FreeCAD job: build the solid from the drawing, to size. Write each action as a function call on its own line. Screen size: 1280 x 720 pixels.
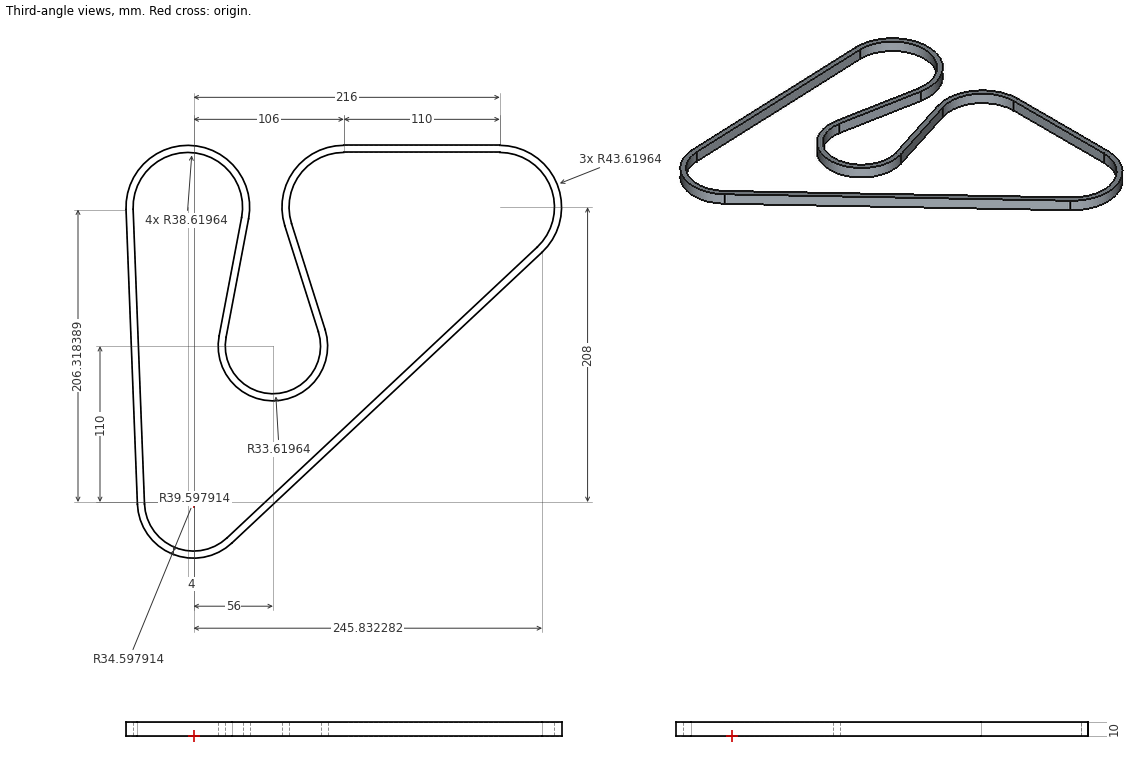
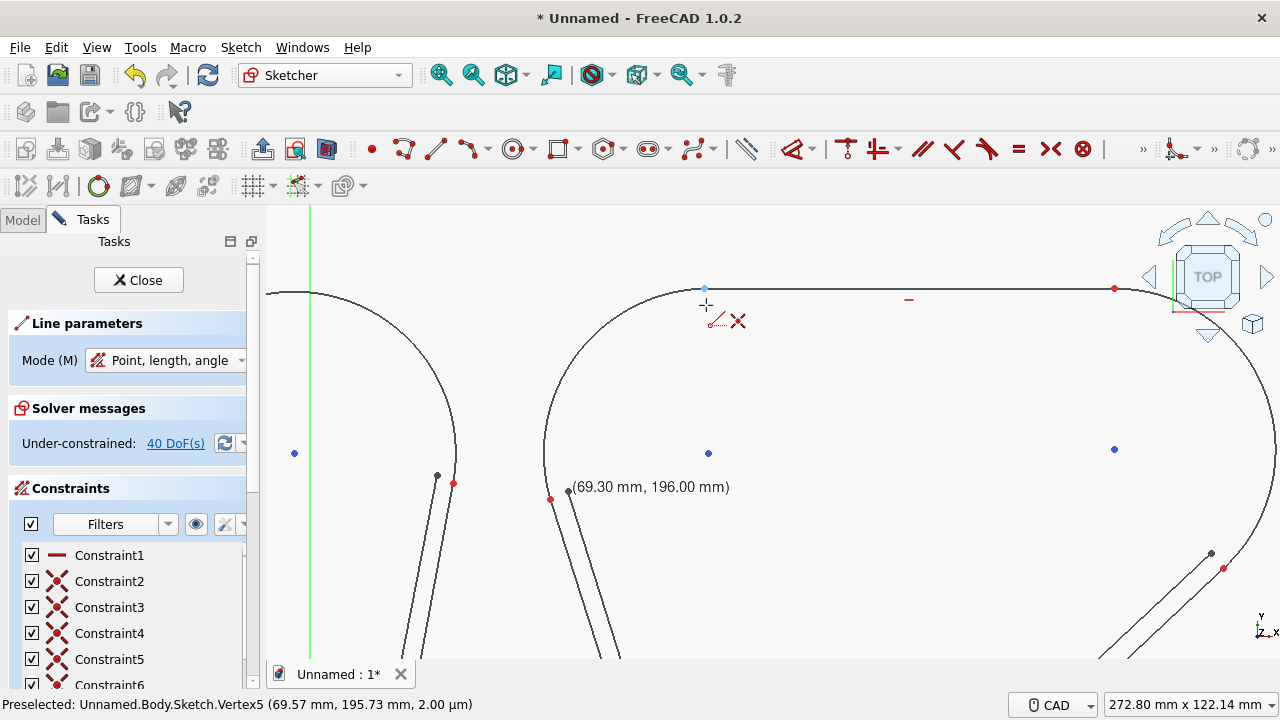
click(704, 304)
click(1113, 304)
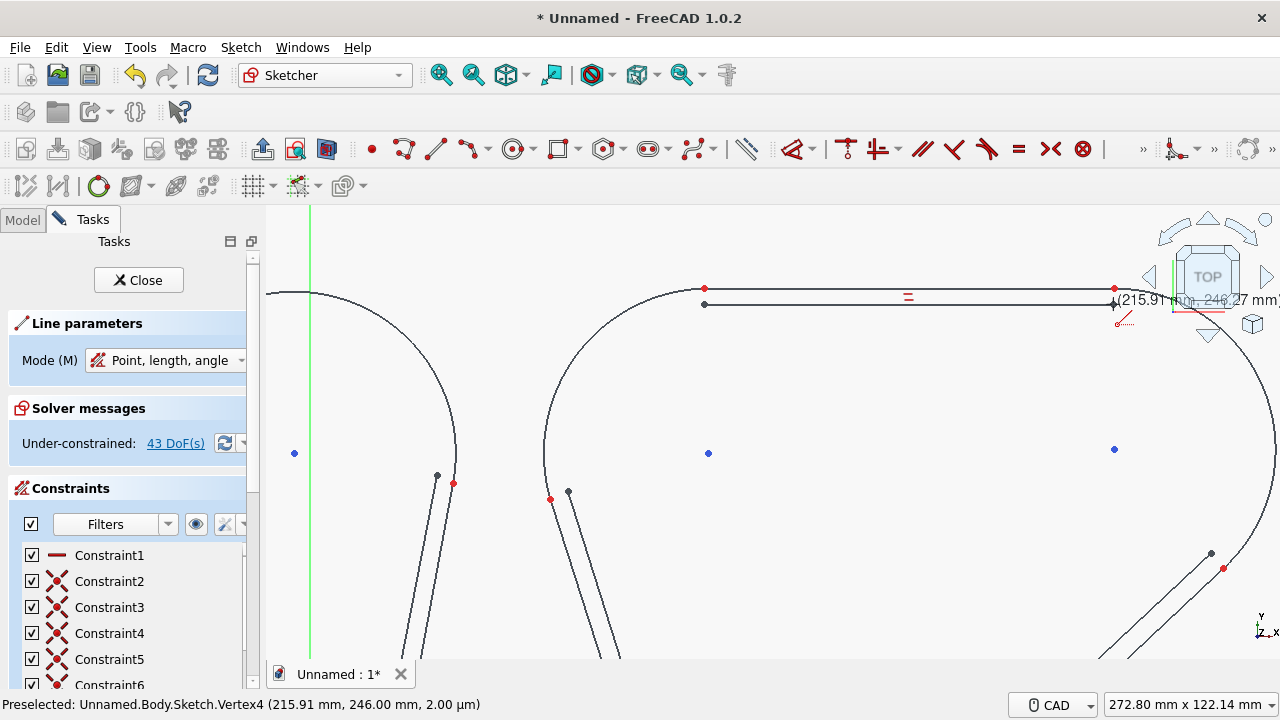
key(g)
key(3)
key(a)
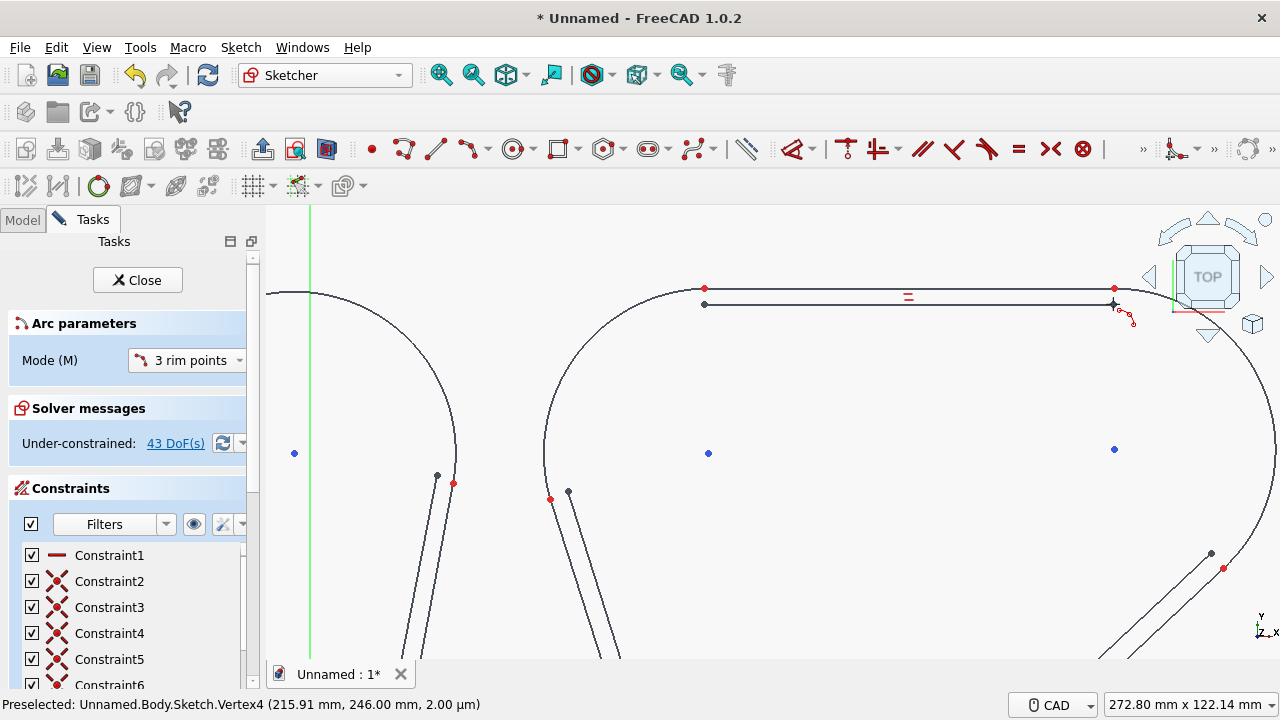
scroll(706, 305, down, 7)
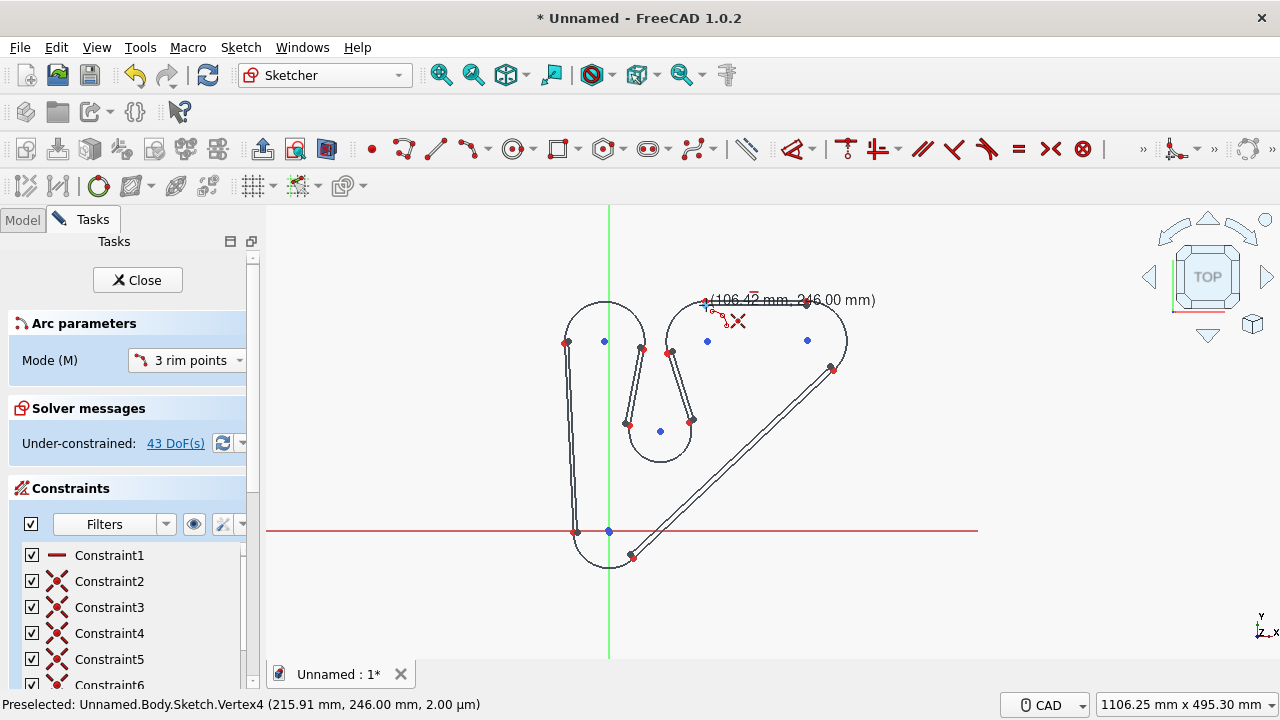
scroll(630, 554, up, 7)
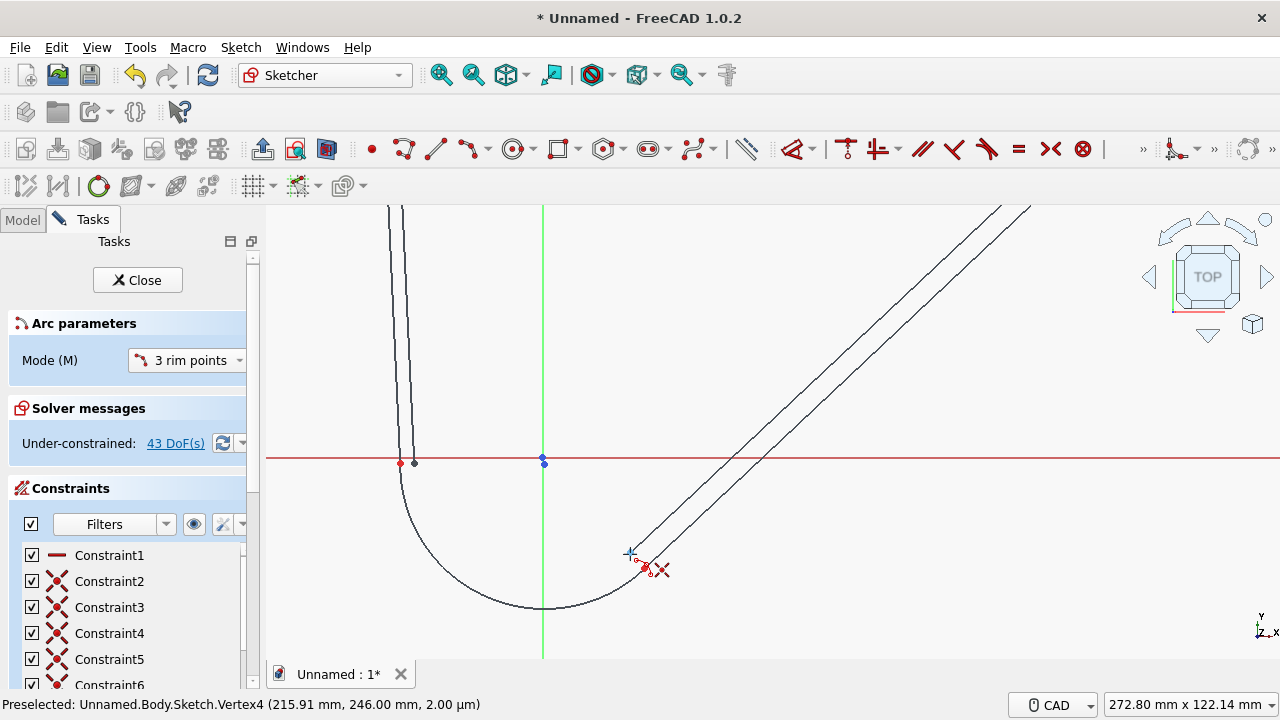
click(631, 552)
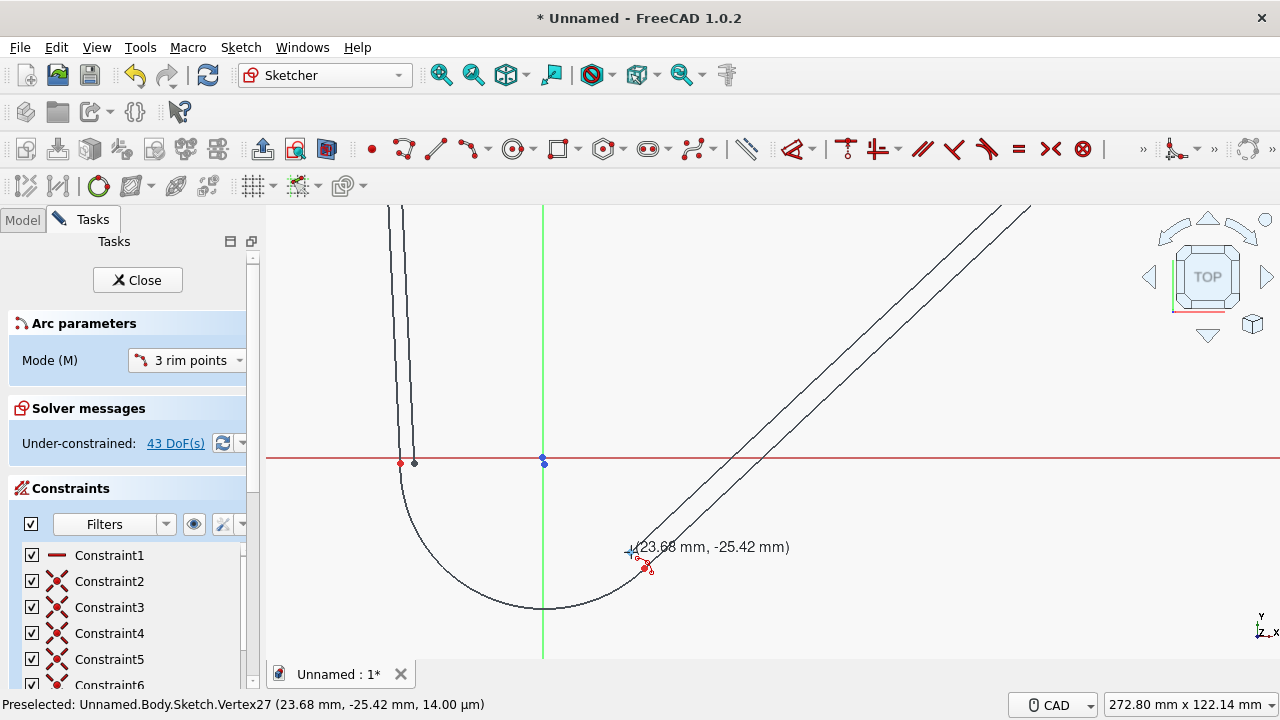
scroll(414, 463, up, 6)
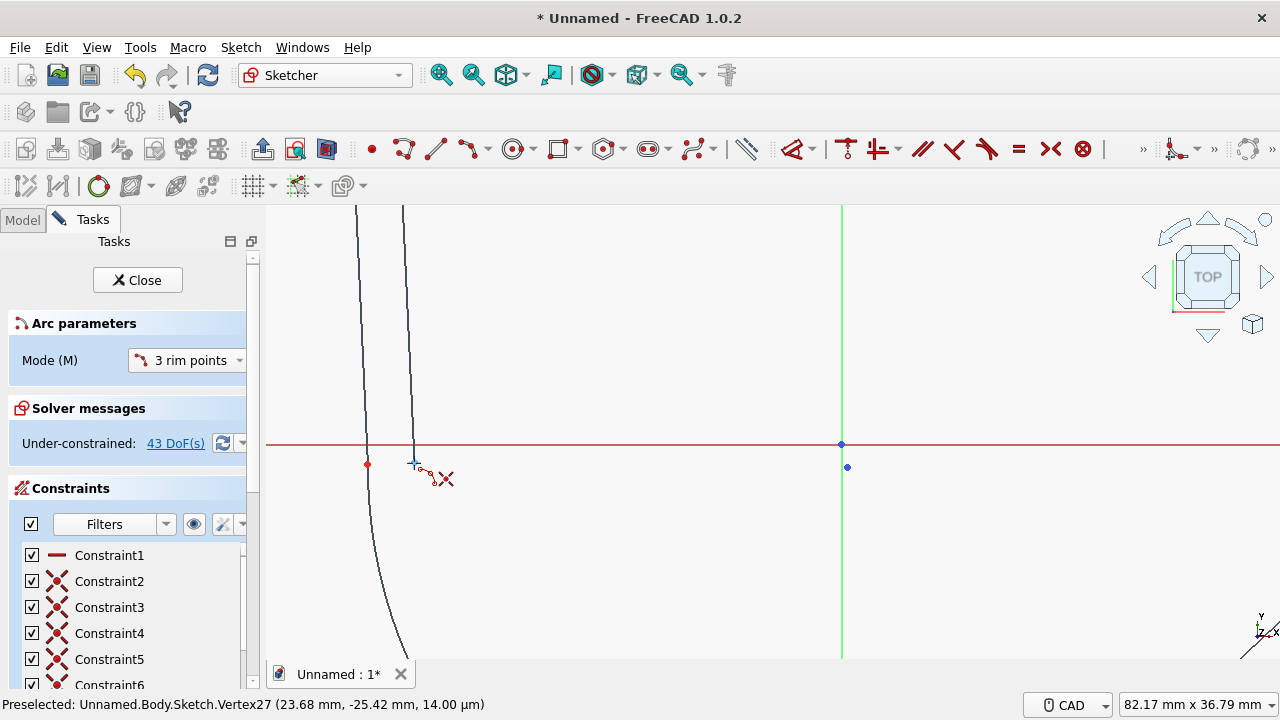
click(415, 462)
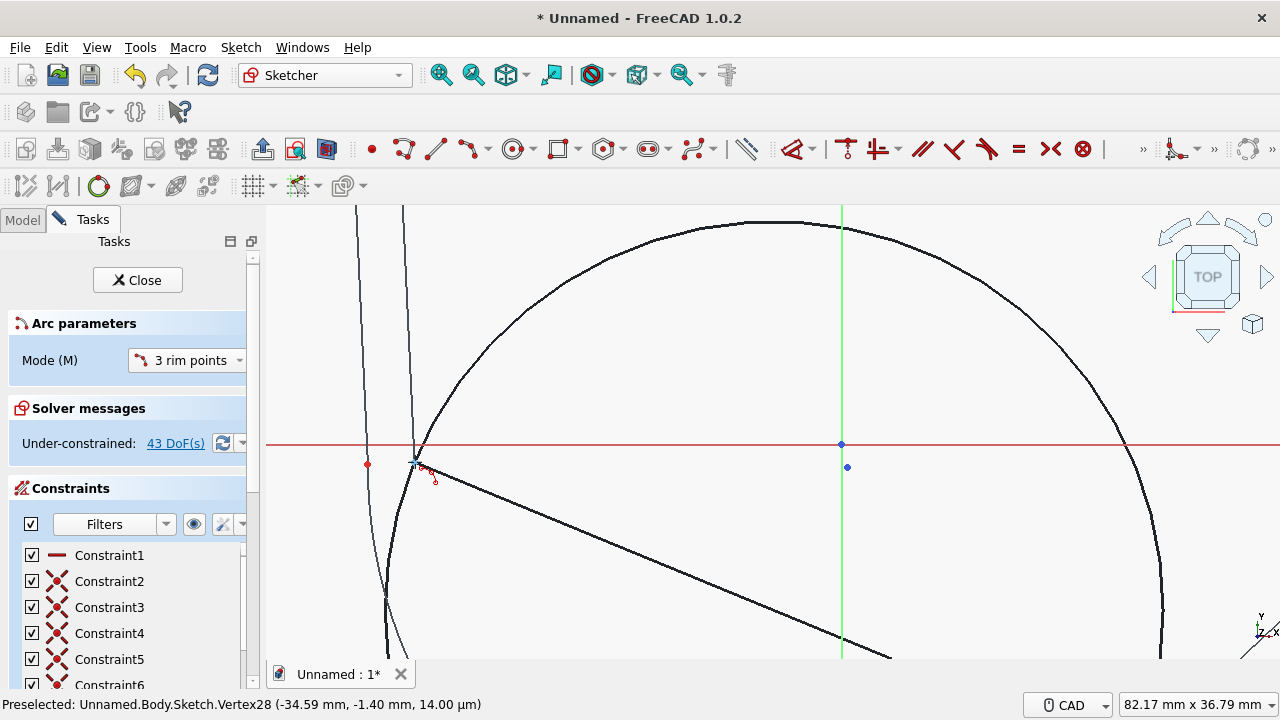
scroll(590, 537, down, 13)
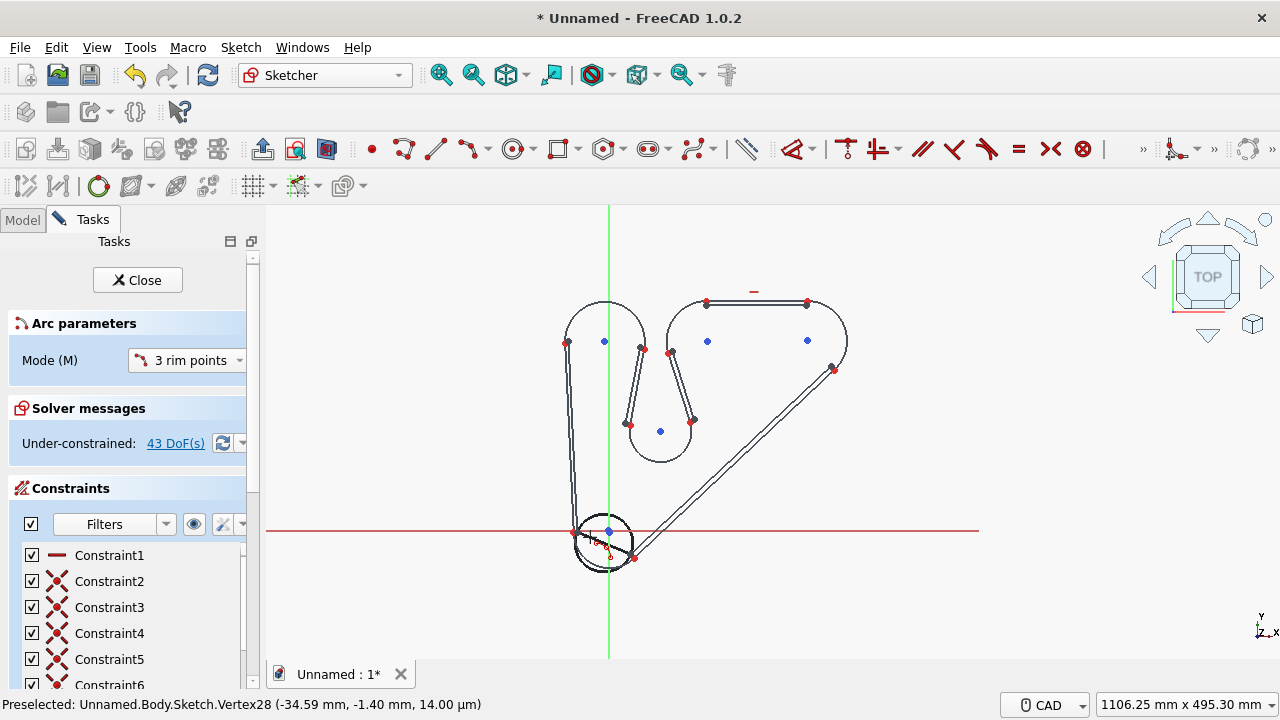
scroll(597, 560, up, 7)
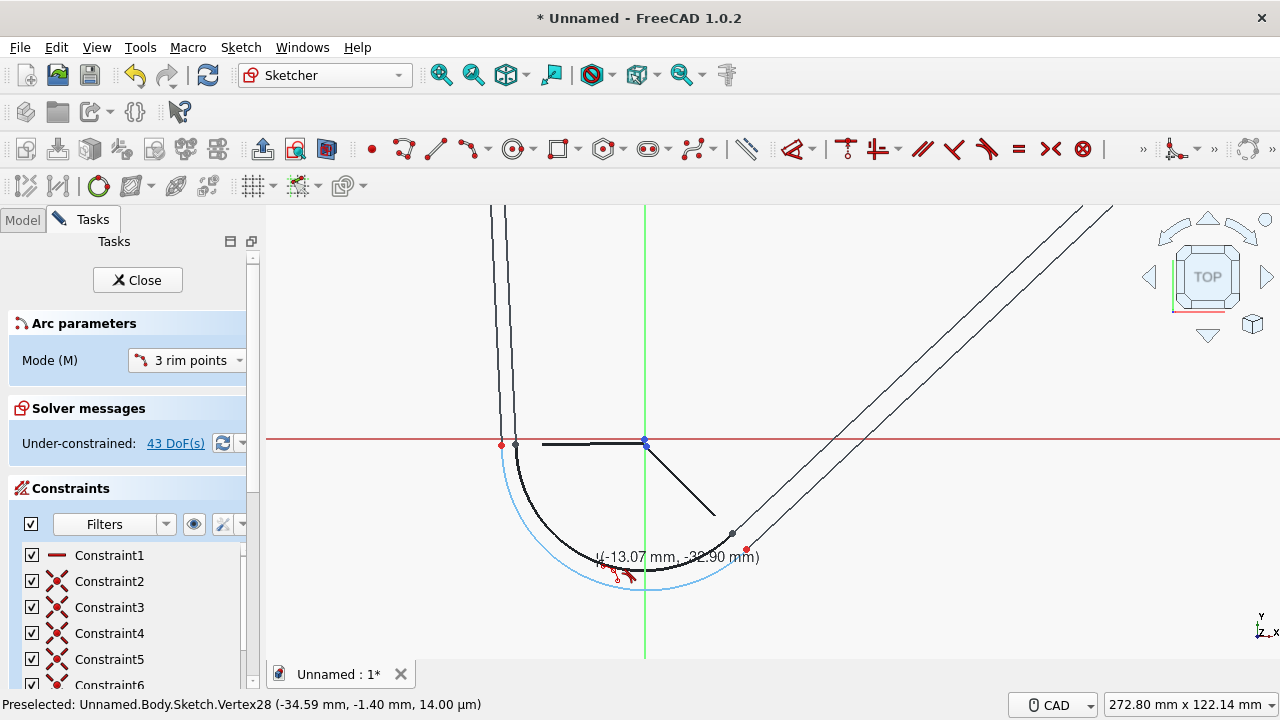
click(596, 558)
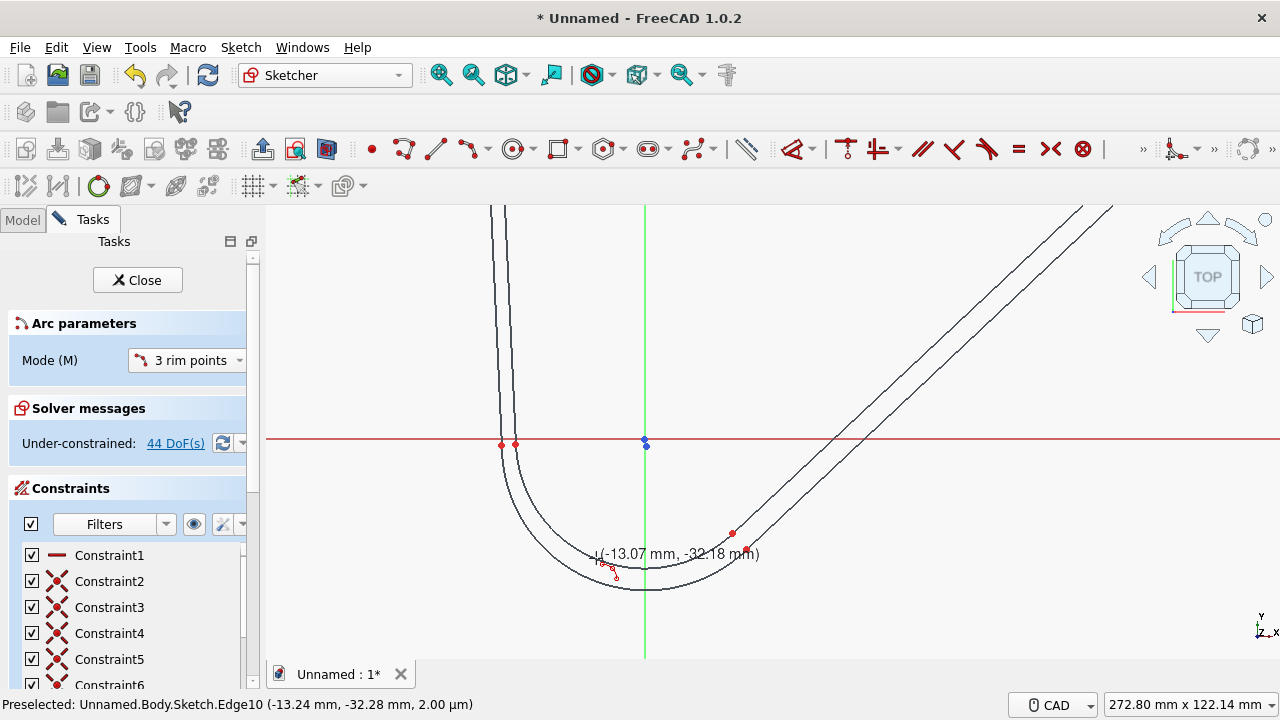
scroll(597, 560, down, 7)